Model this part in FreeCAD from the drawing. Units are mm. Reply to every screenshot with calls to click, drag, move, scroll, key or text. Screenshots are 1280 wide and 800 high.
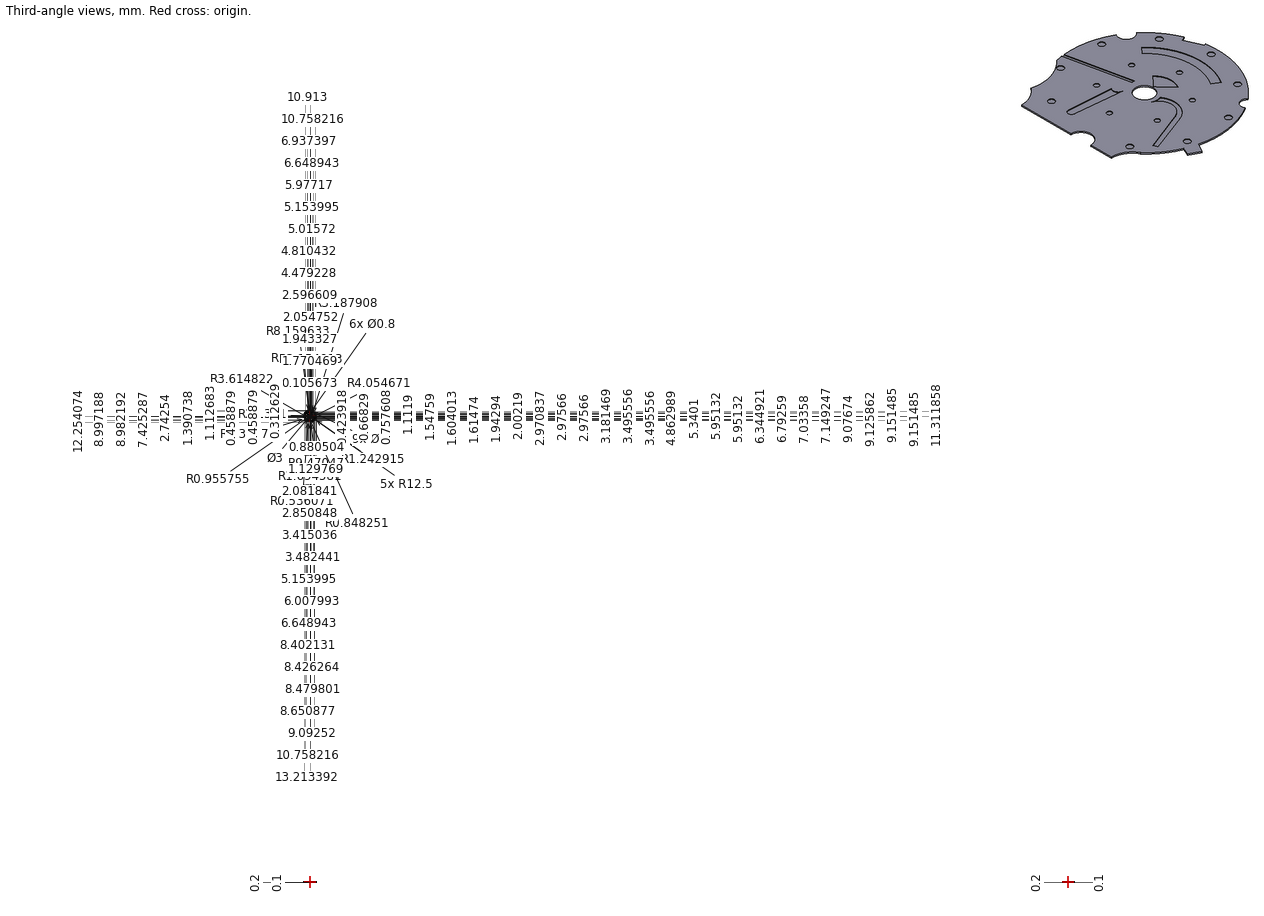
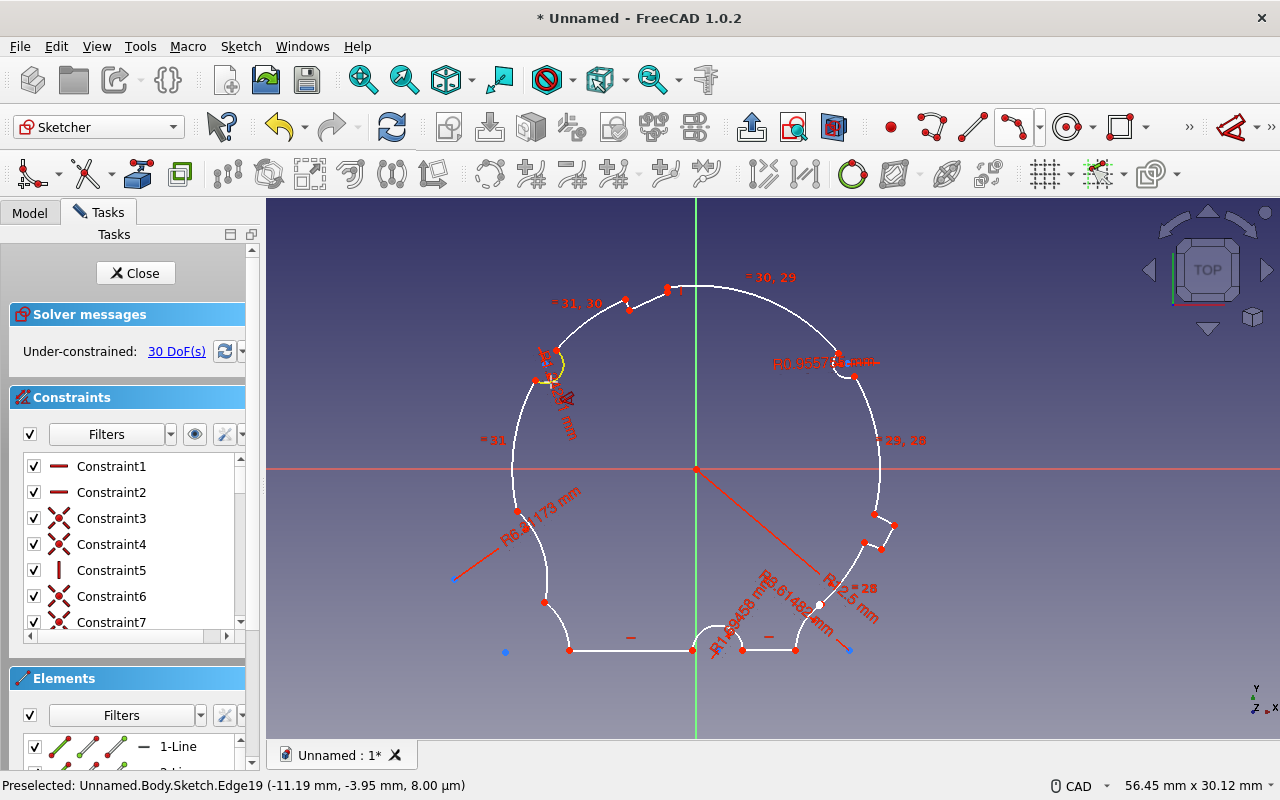
click(567, 634)
click(598, 625)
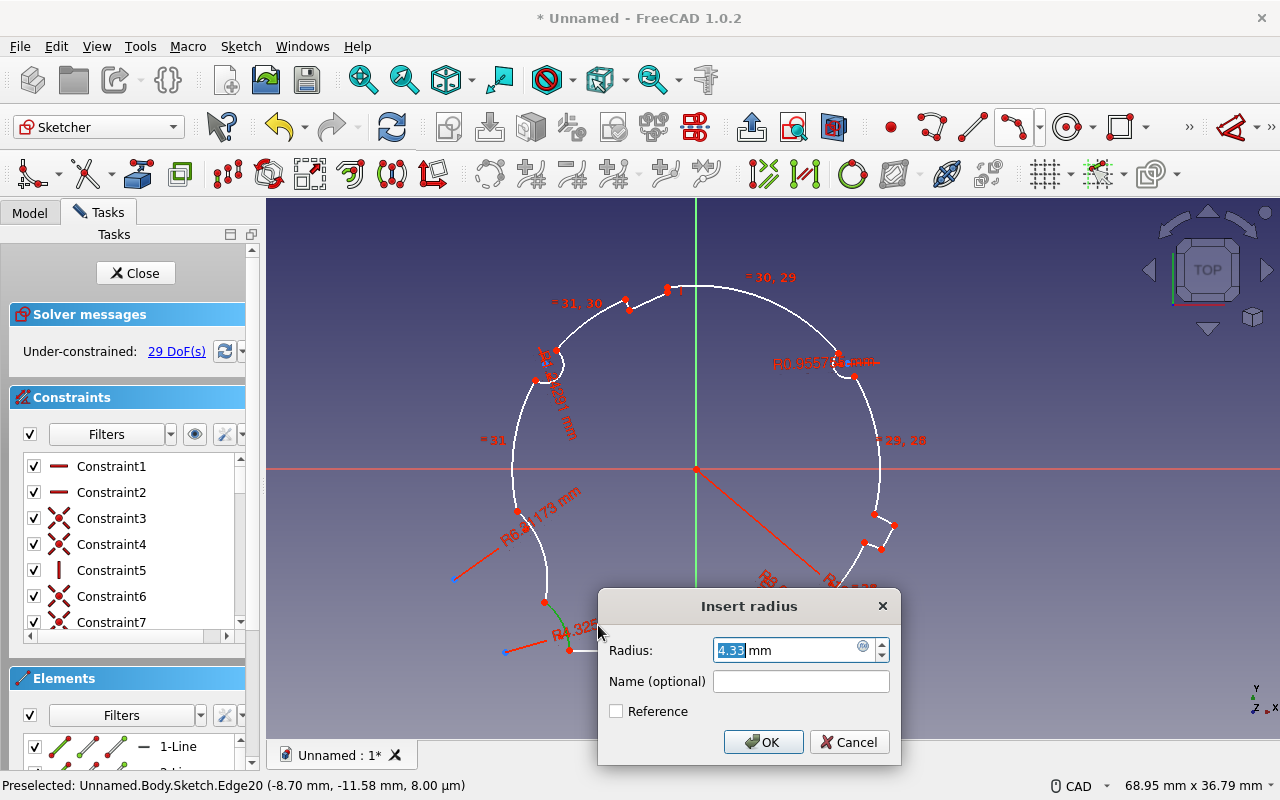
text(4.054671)
key(Return)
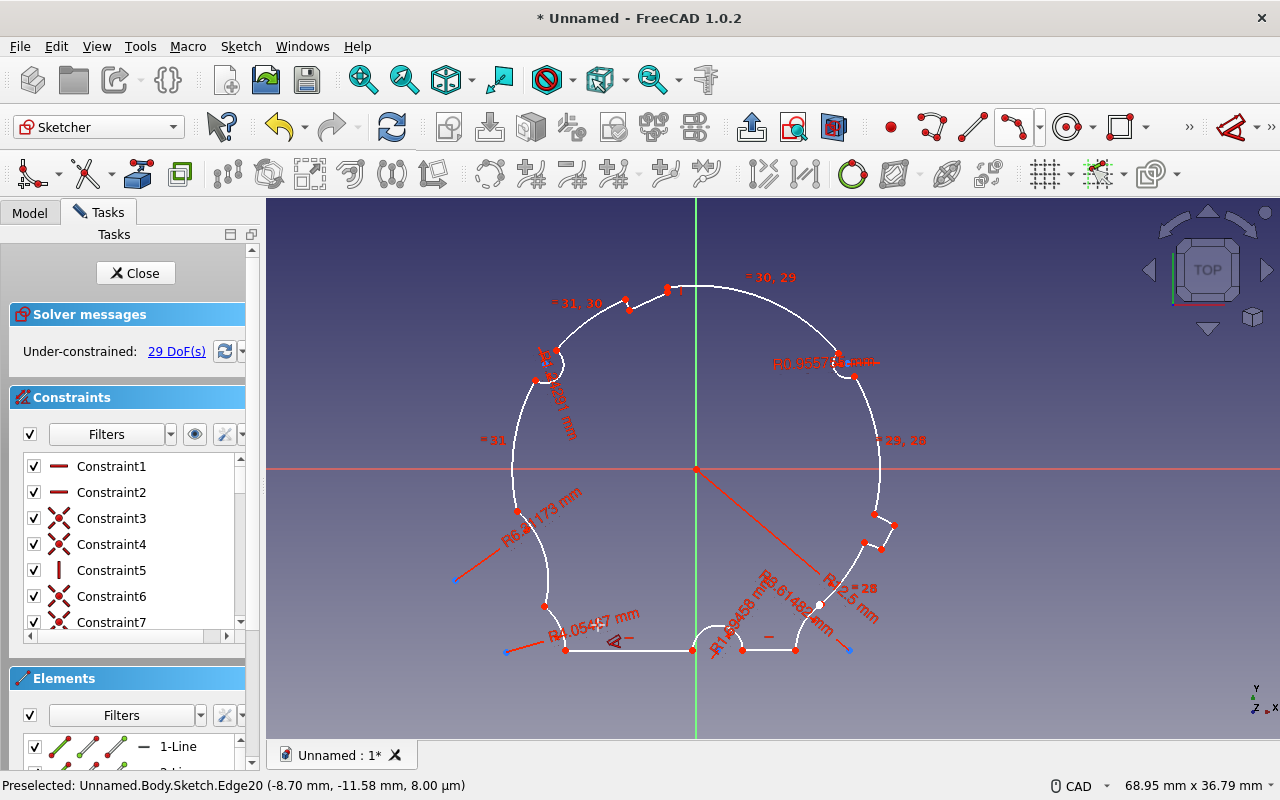
click(882, 549)
click(916, 509)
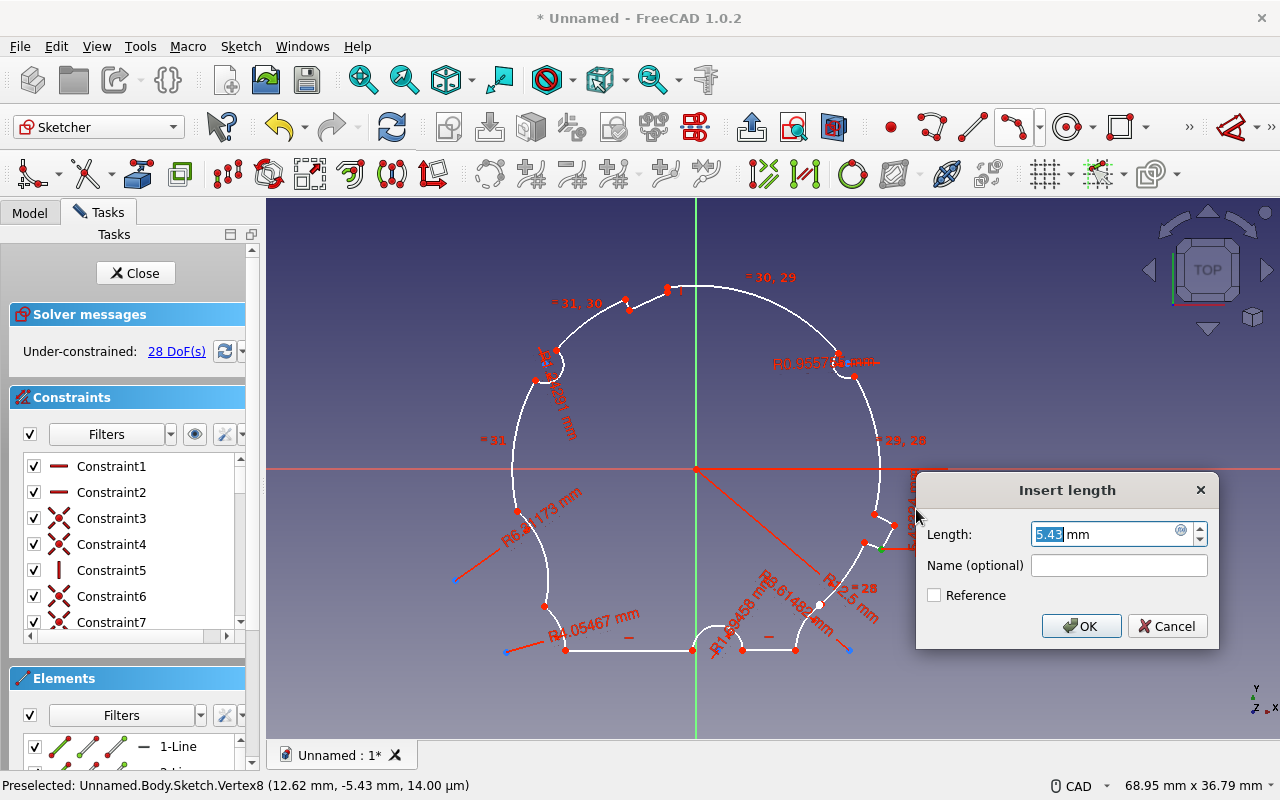
text(5.3401)
key(Return)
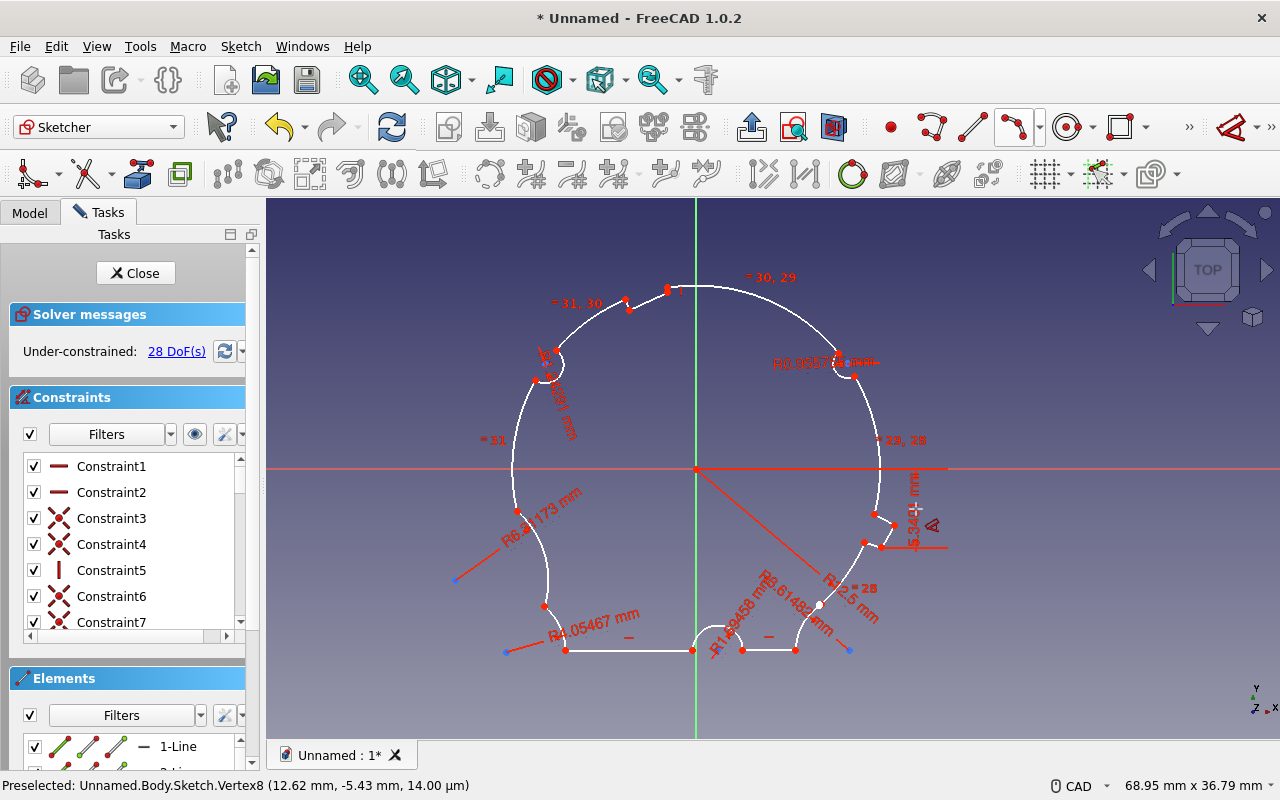
click(535, 380)
click(616, 346)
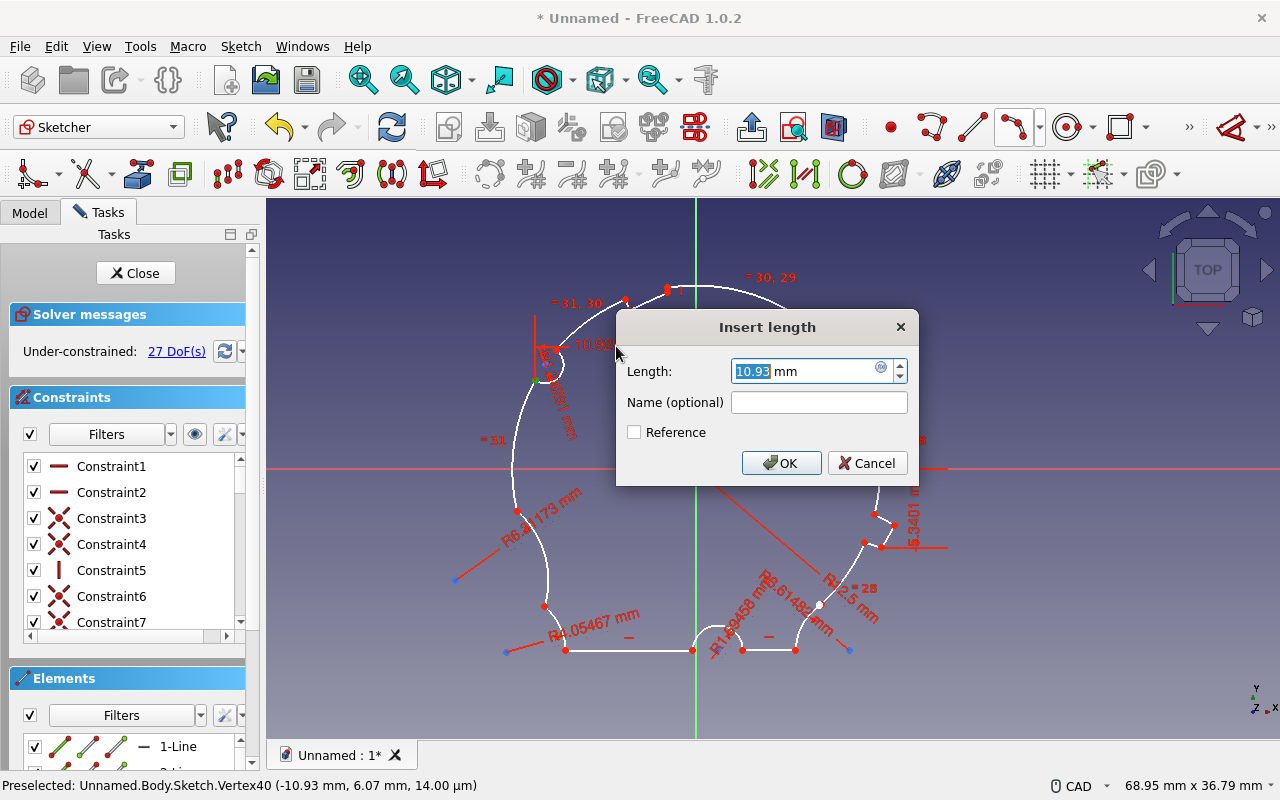
text(10.913)
key(Return)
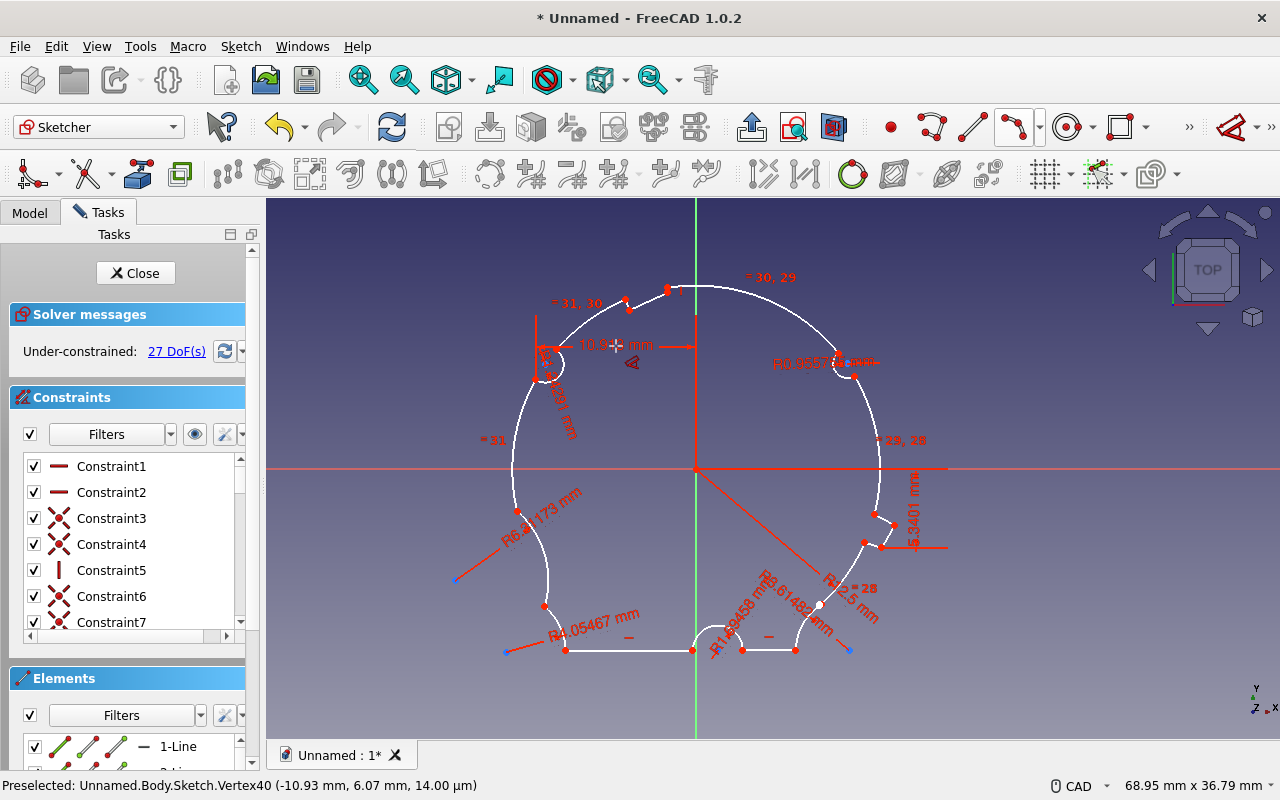
click(604, 651)
click(629, 685)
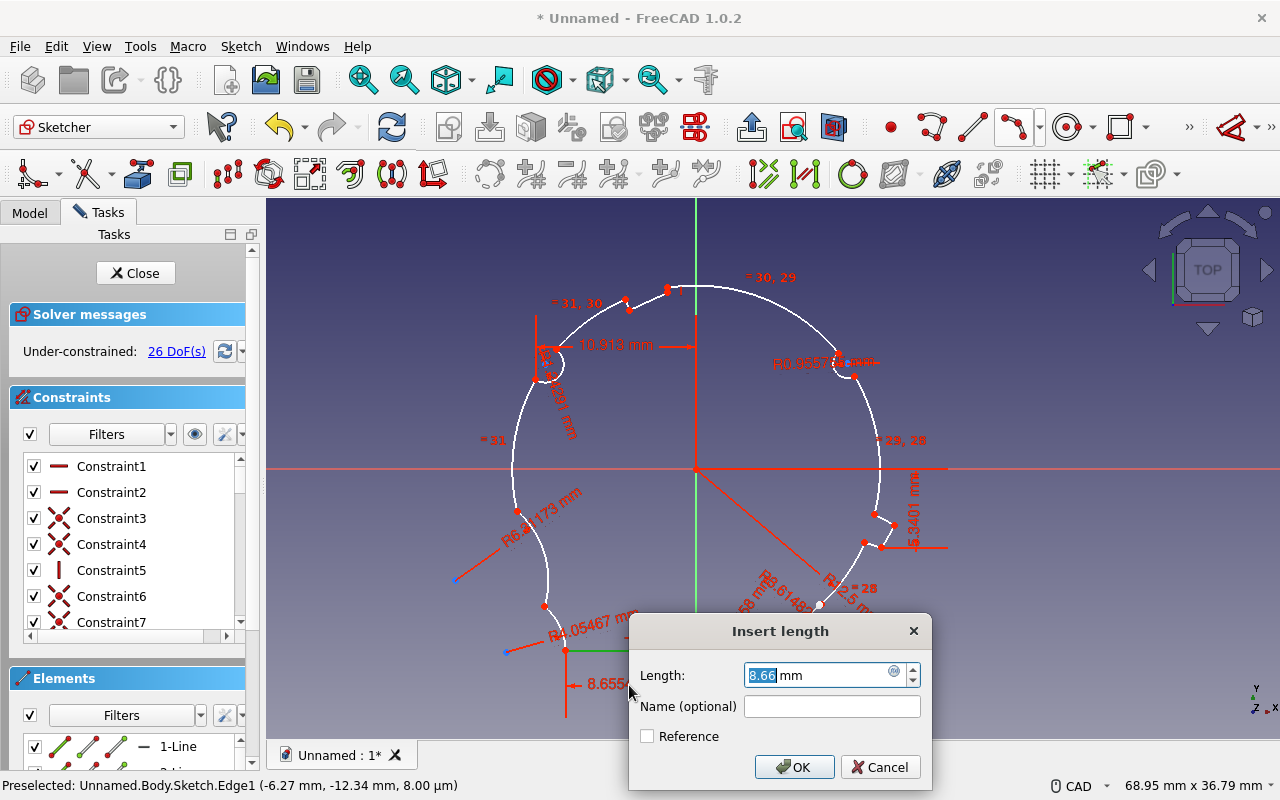
text(8.402131)
key(Return)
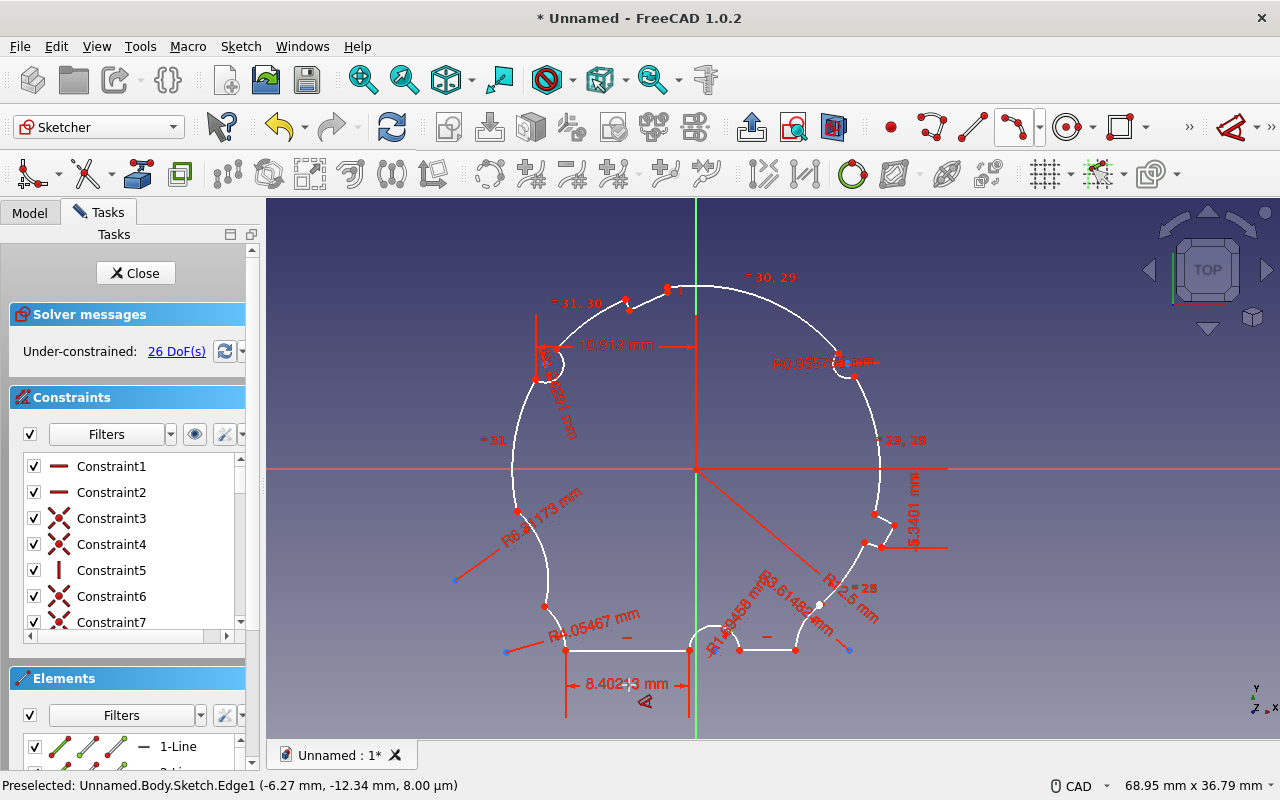
click(756, 650)
click(768, 684)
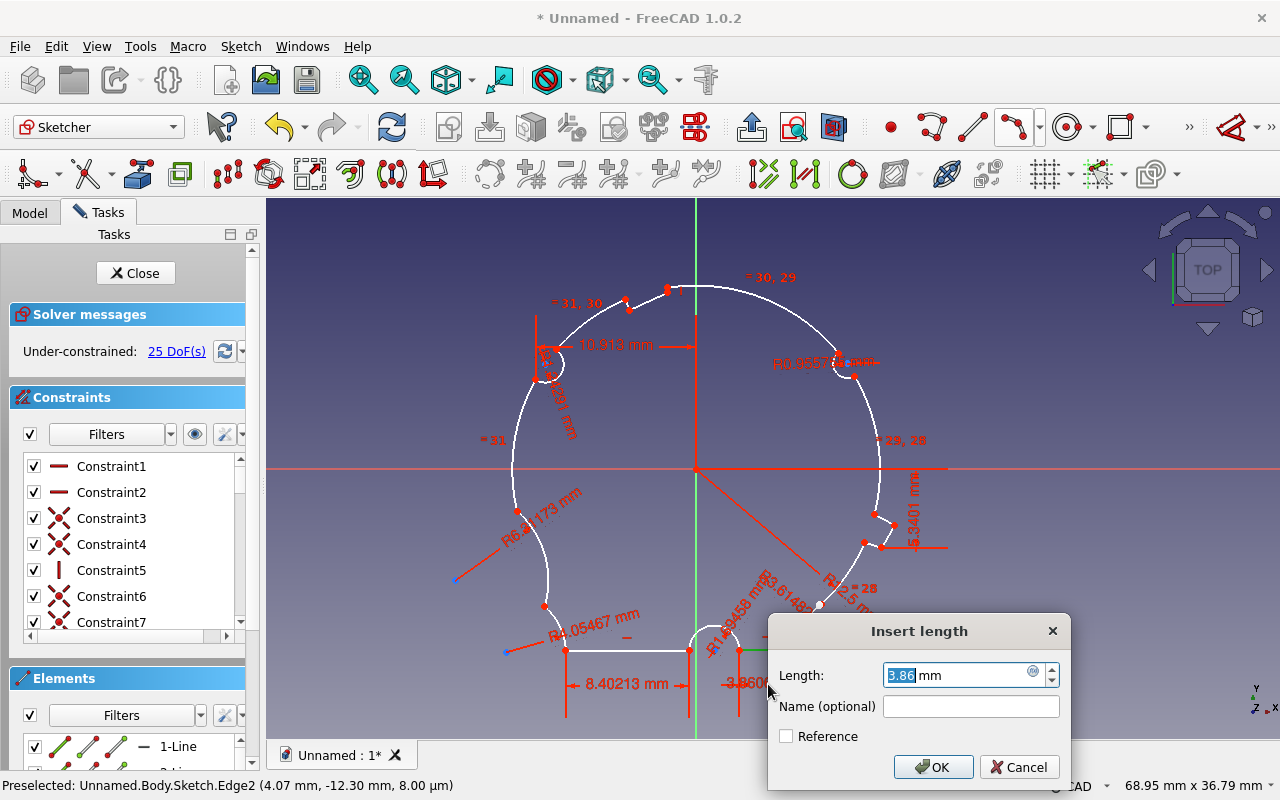
text(3.482441)
key(Return)